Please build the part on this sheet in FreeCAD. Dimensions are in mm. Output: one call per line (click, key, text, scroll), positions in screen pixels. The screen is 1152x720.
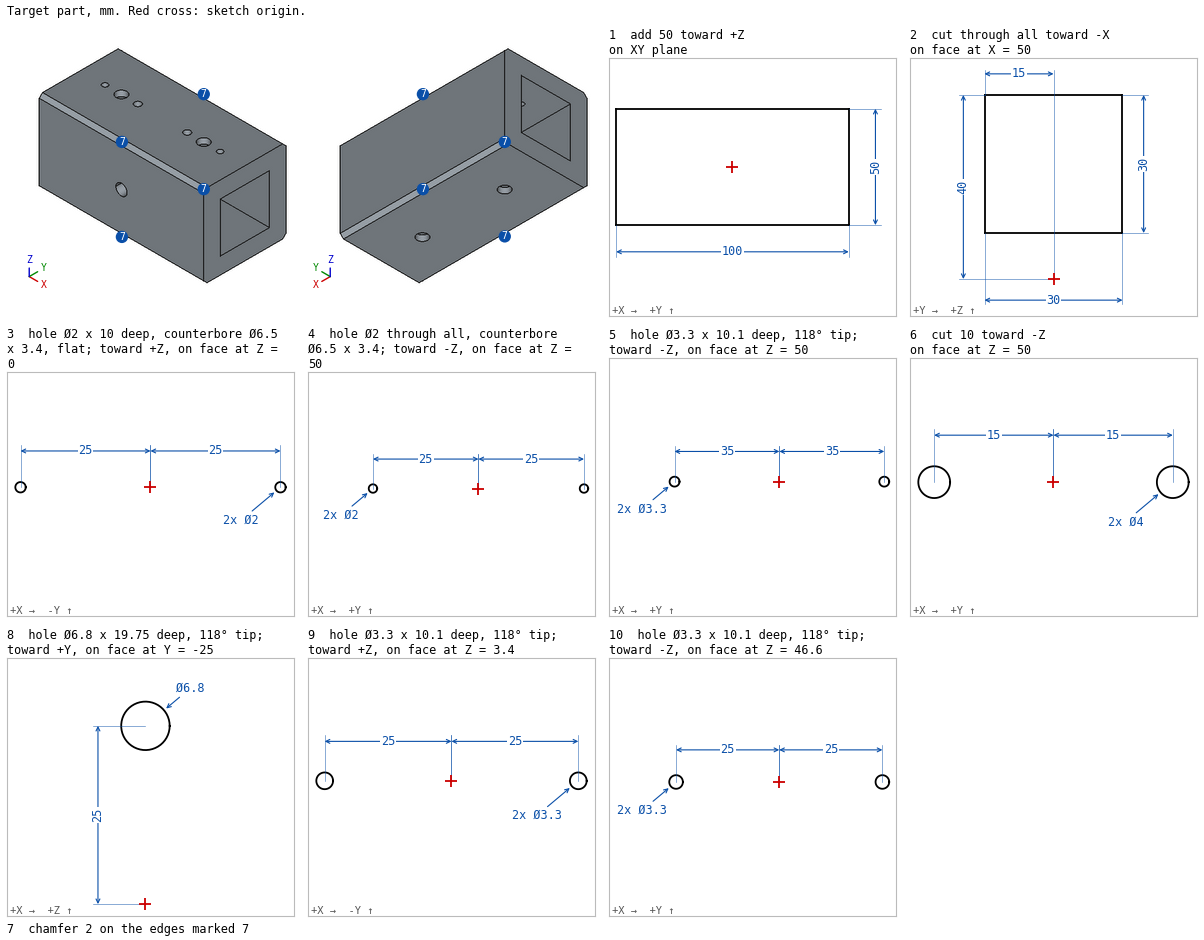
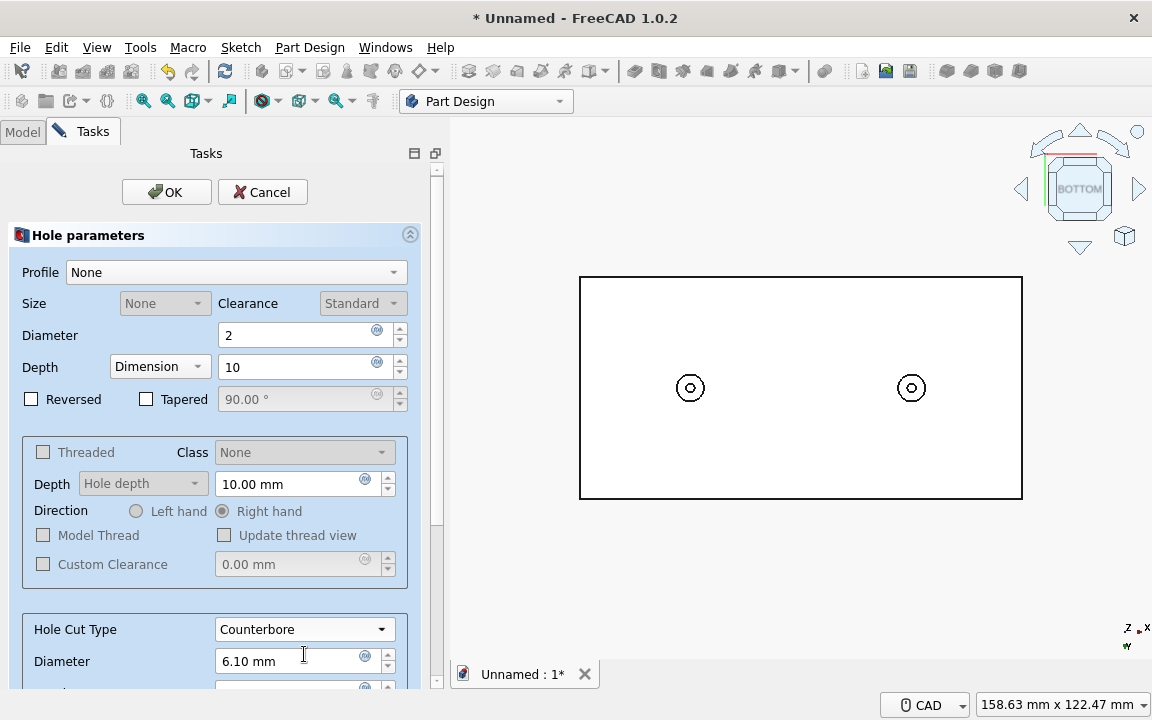
triple_click(298, 661)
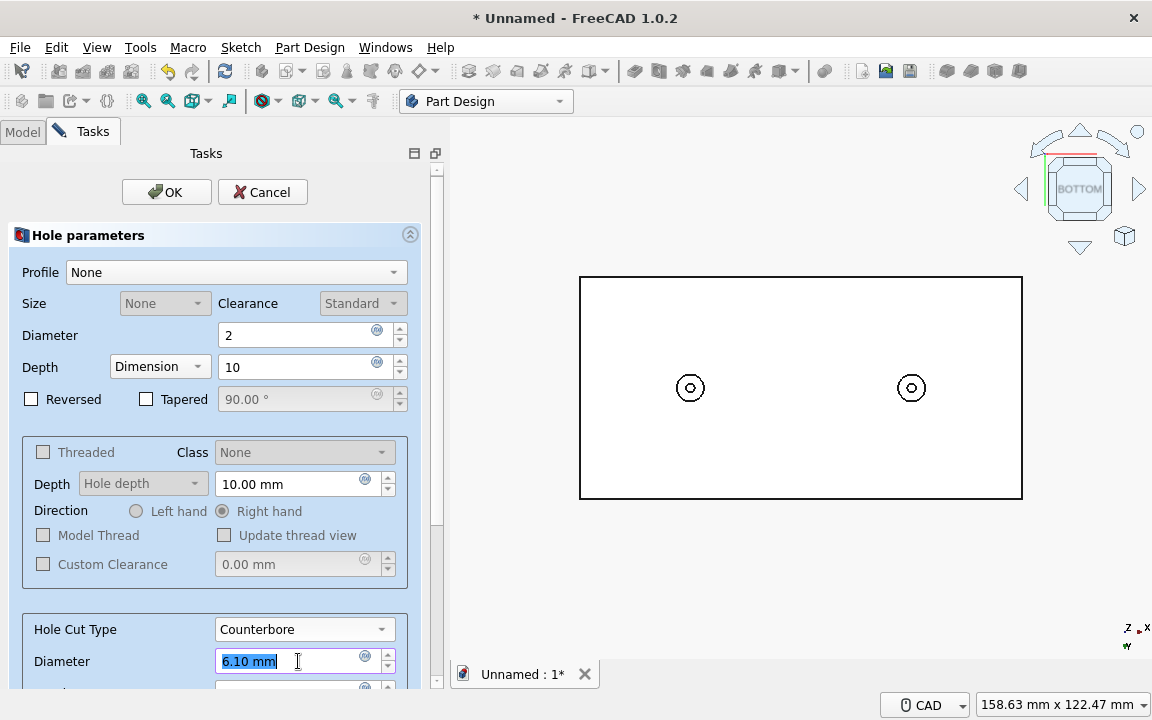
text(6.5)
key(Tab)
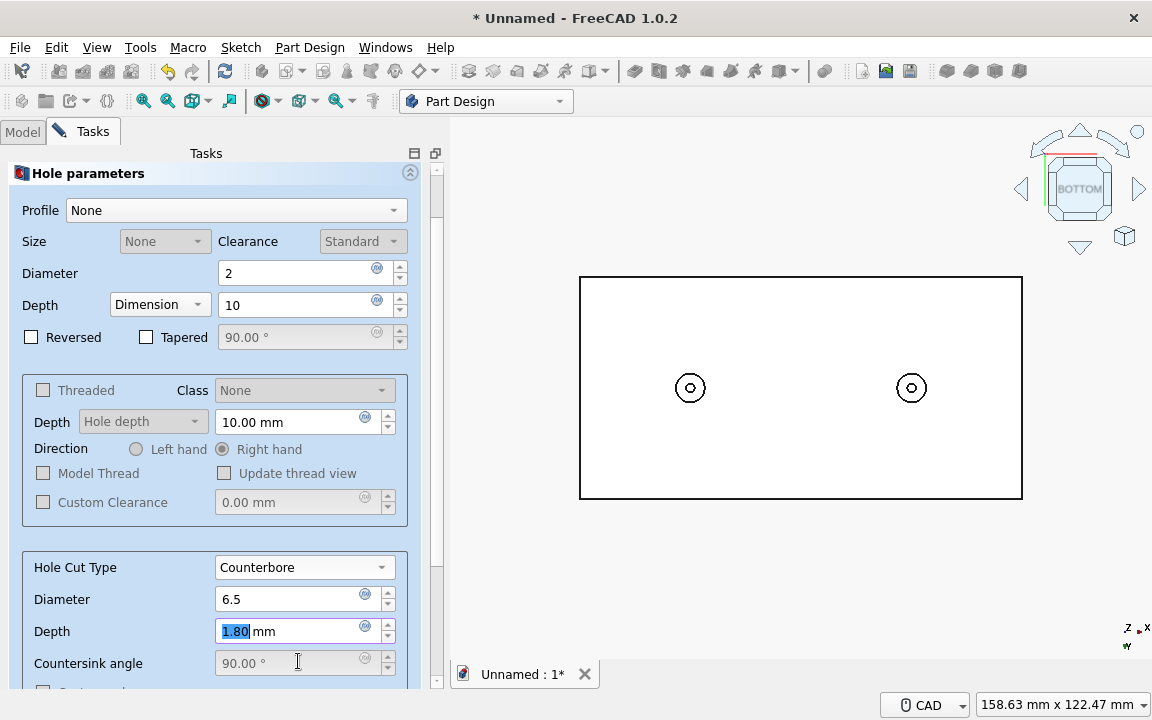
text(3.4)
key(Tab)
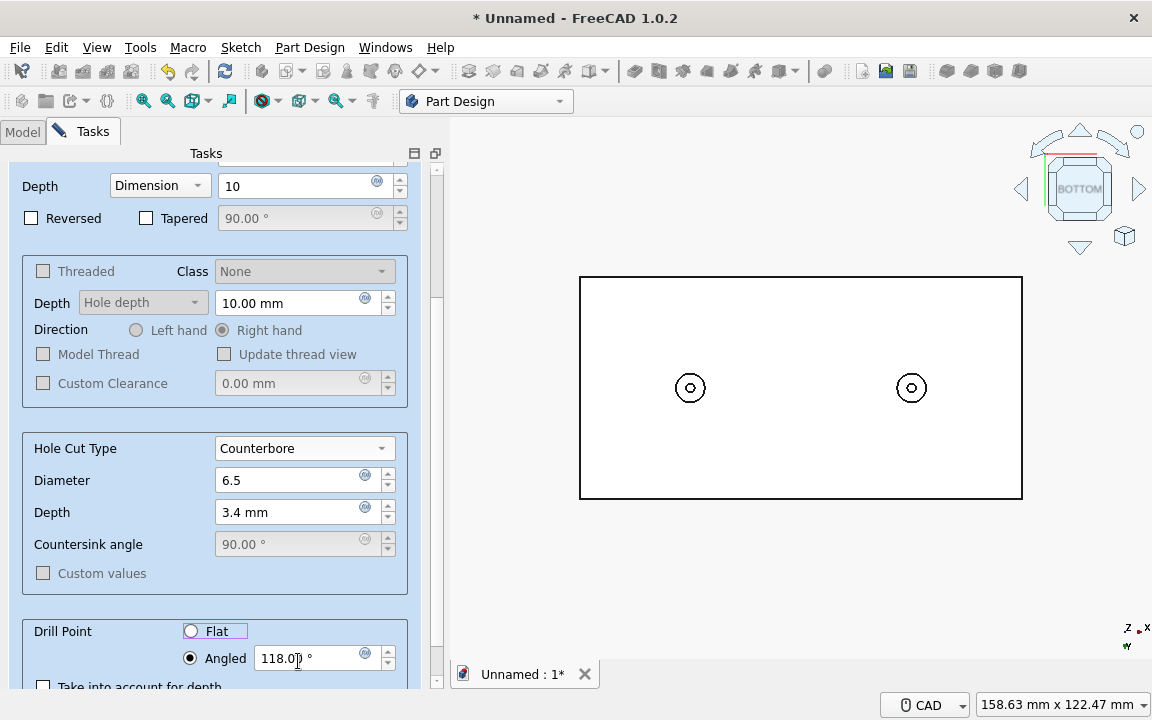
click(191, 631)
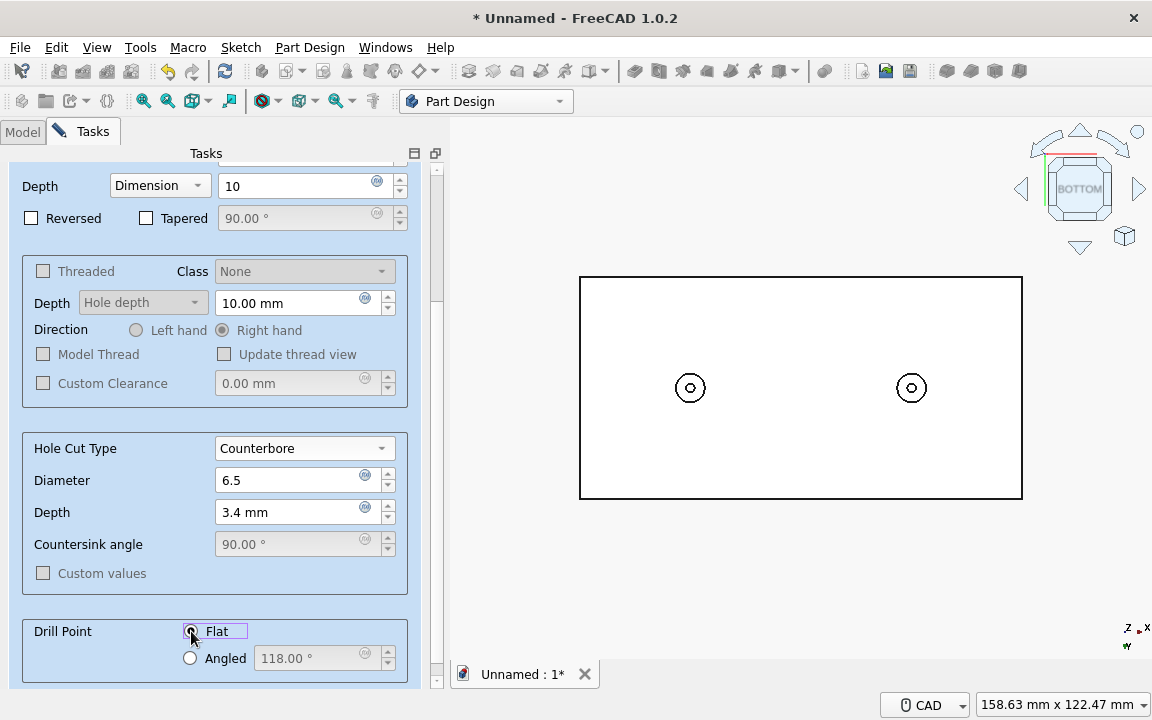
scroll(437, 426, up, 4)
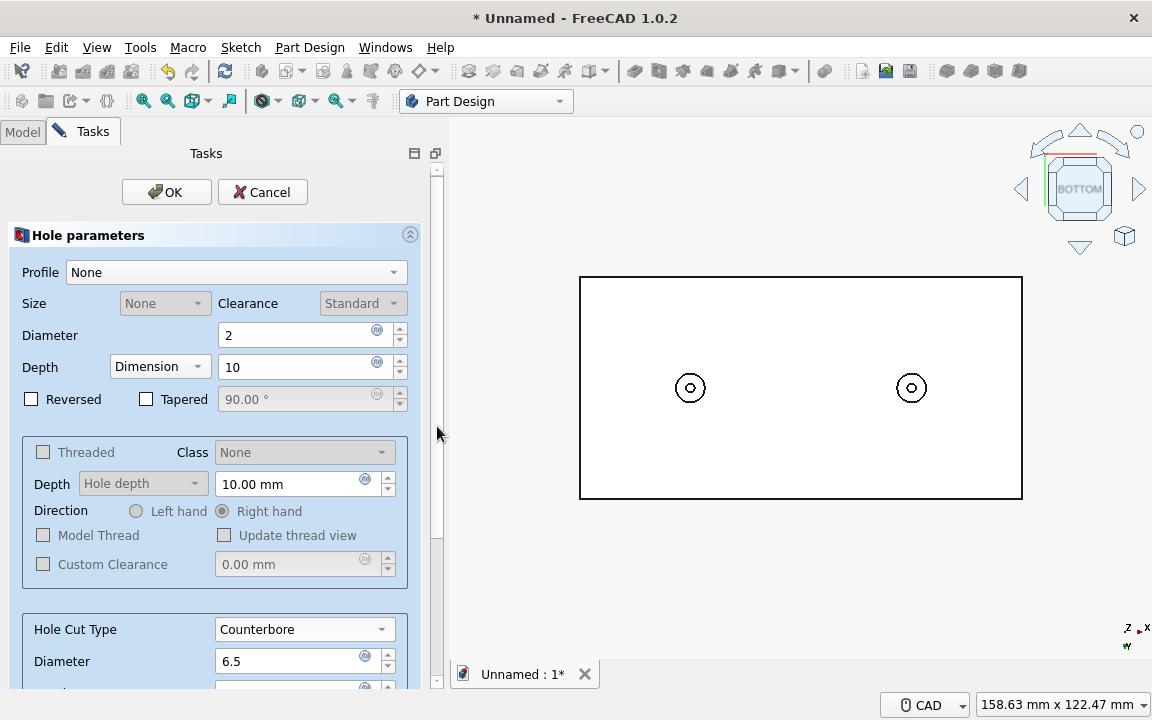
click(167, 192)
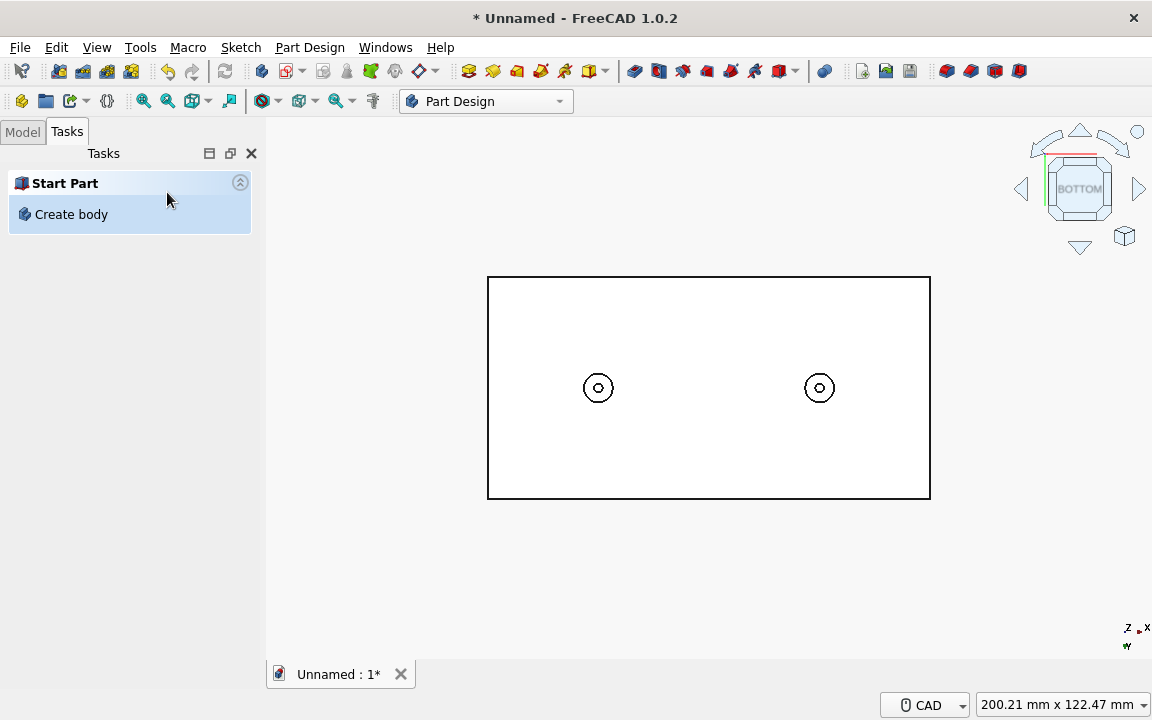
key(0)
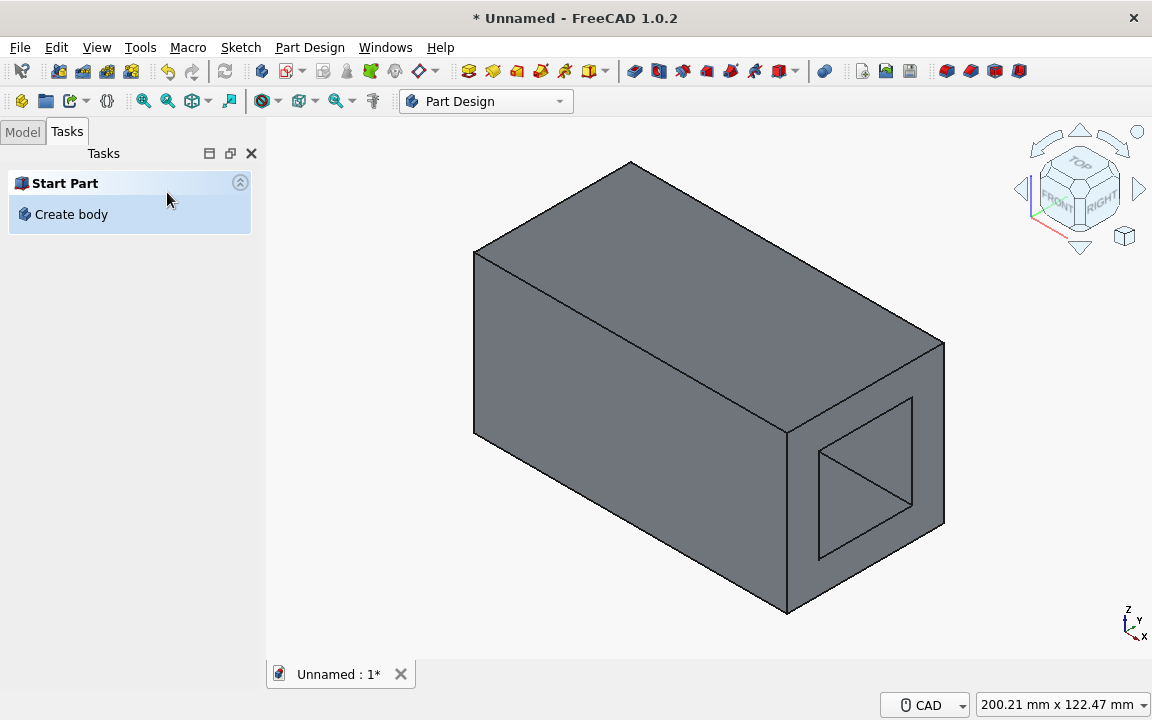
click(754, 322)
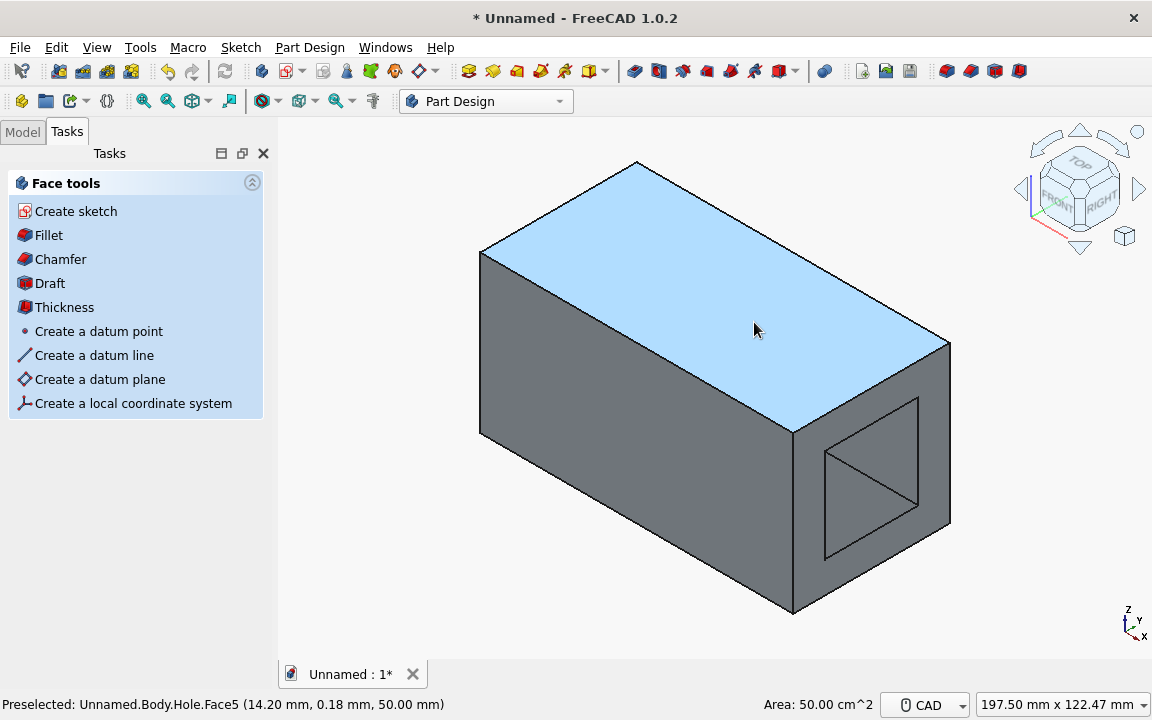
click(286, 72)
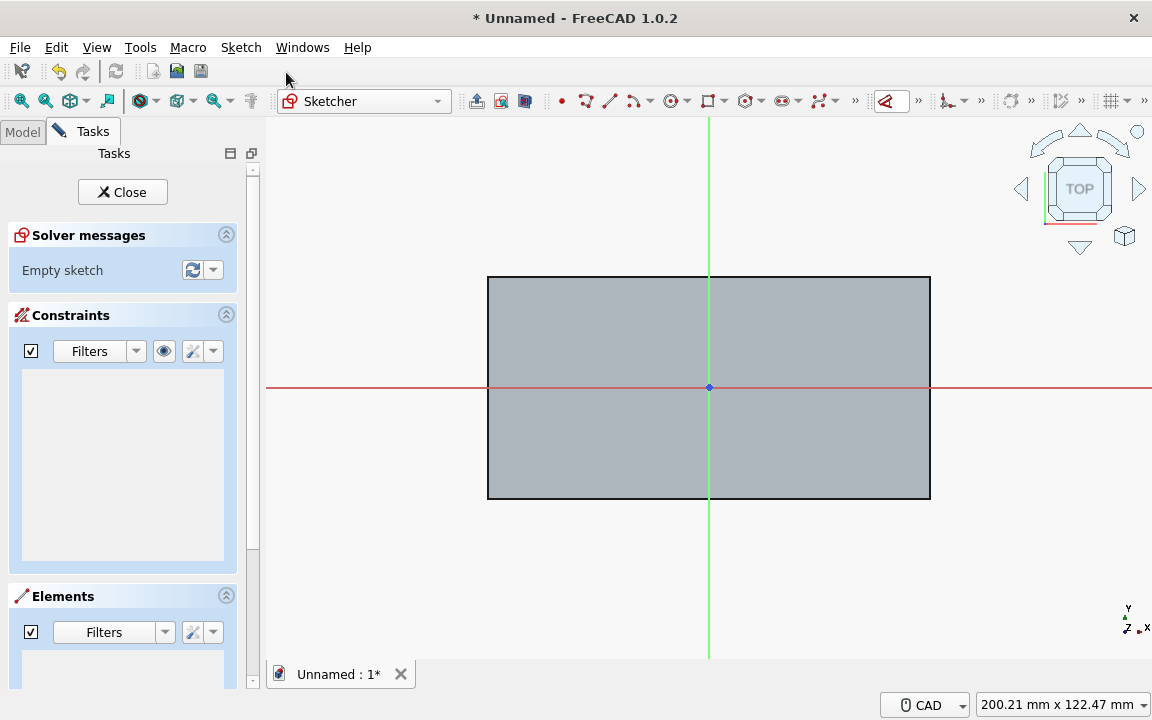
scroll(765, 388, up, 4)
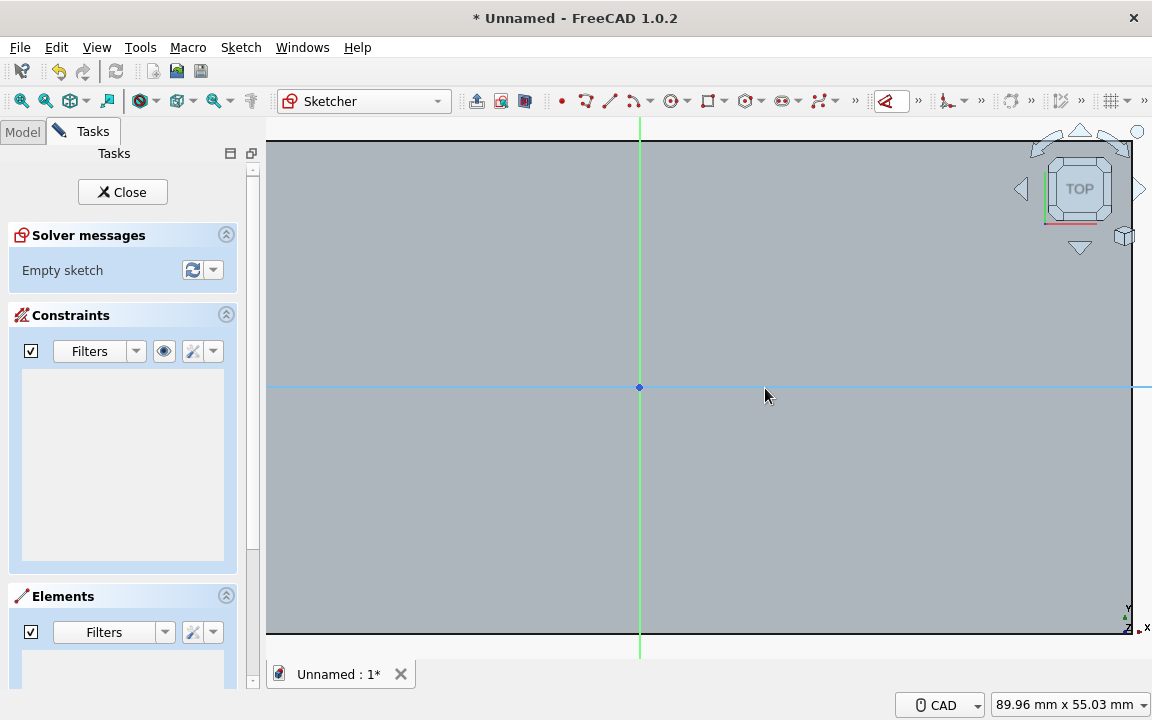
click(672, 102)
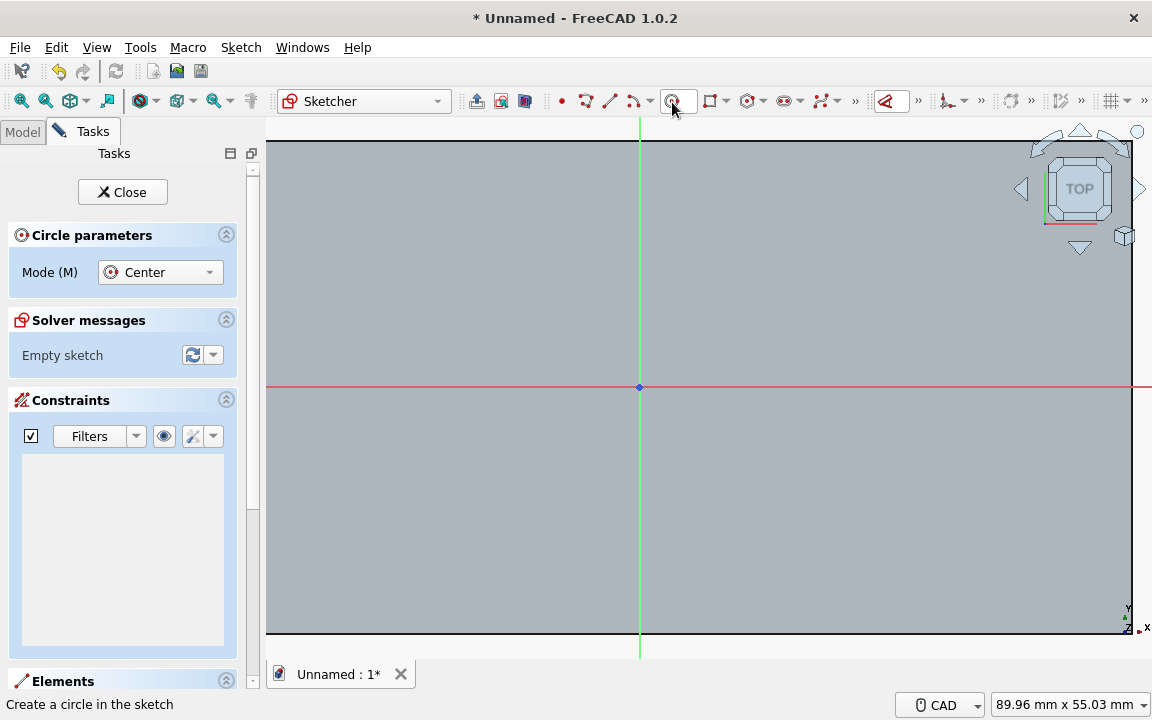
scroll(393, 387, up, 5)